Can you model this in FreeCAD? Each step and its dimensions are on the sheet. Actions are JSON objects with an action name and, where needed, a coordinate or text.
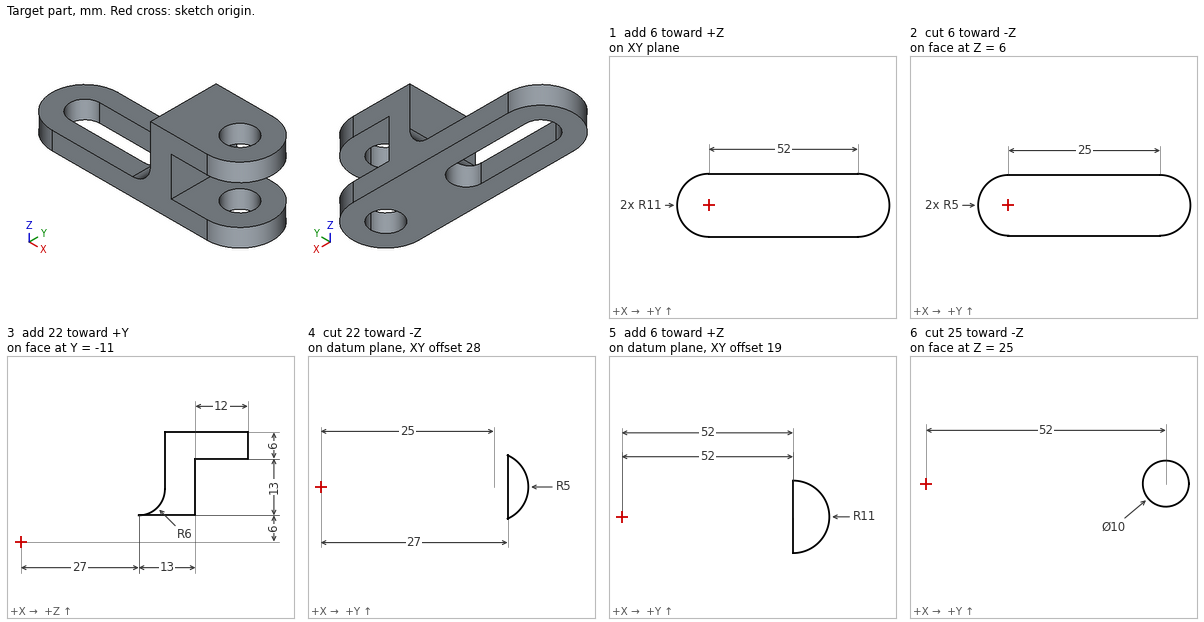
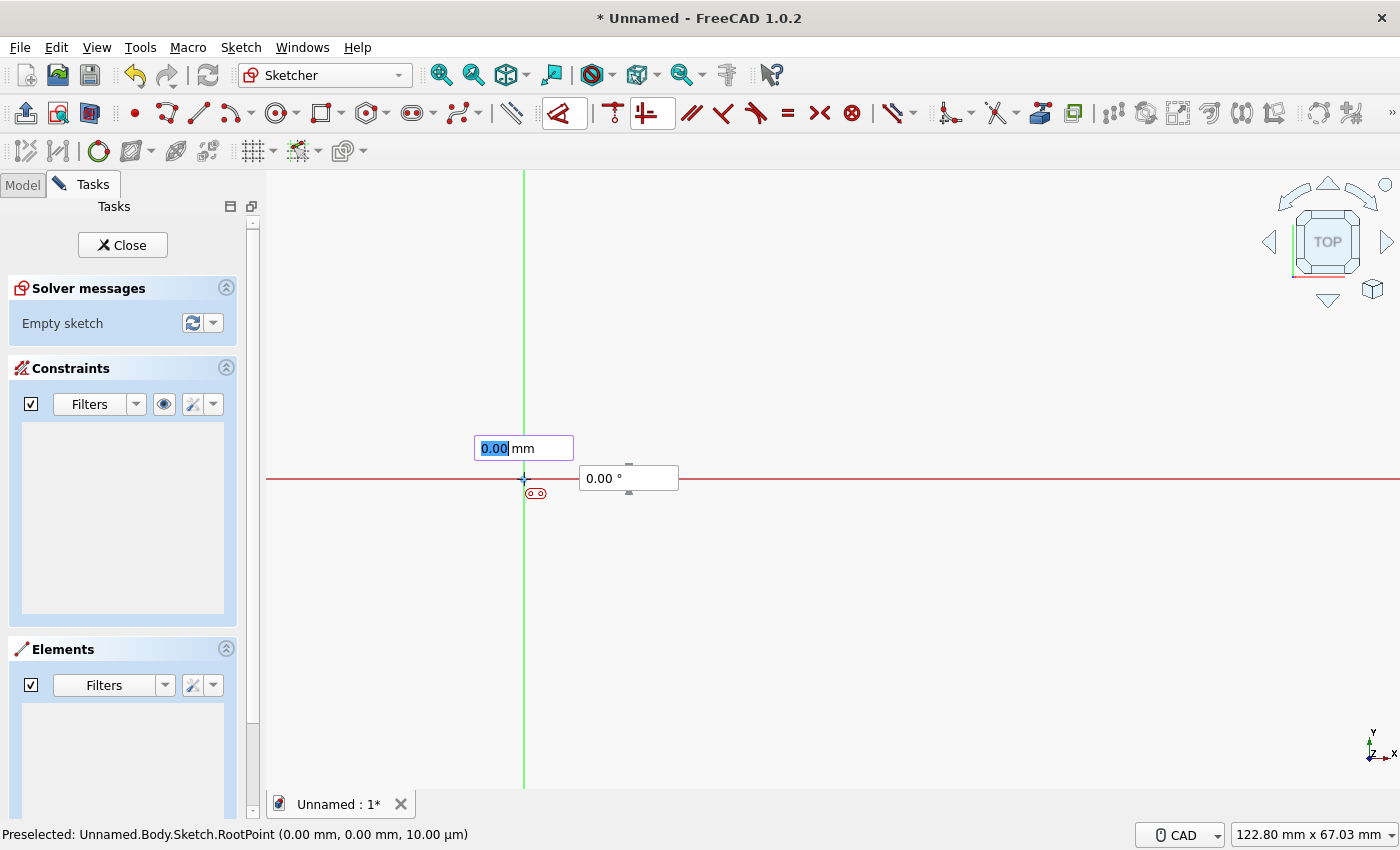
{"action": "left_click", "coordinate": [1004, 470]}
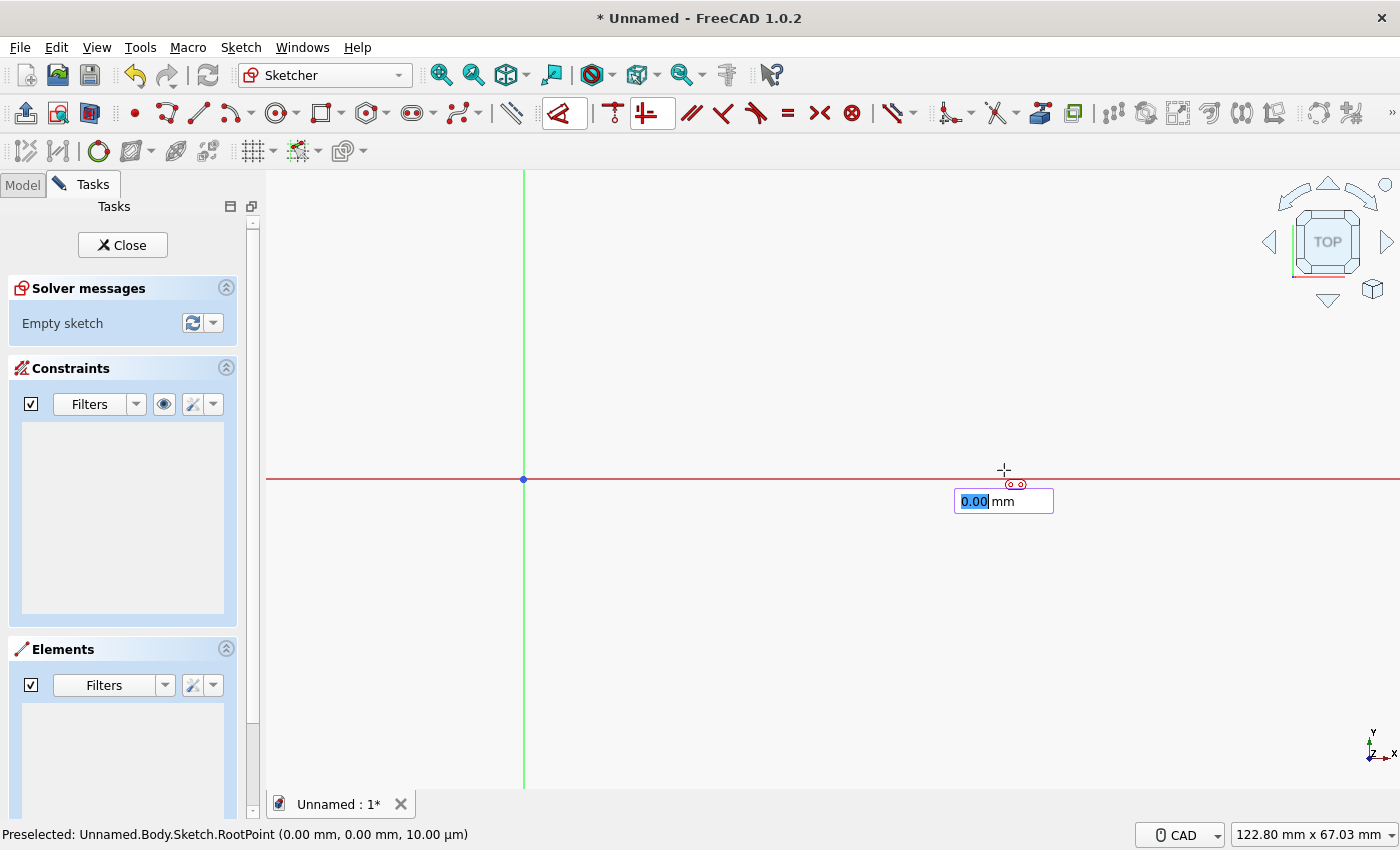
{"action": "left_click", "coordinate": [764, 377]}
{"action": "key", "text": "Escape"}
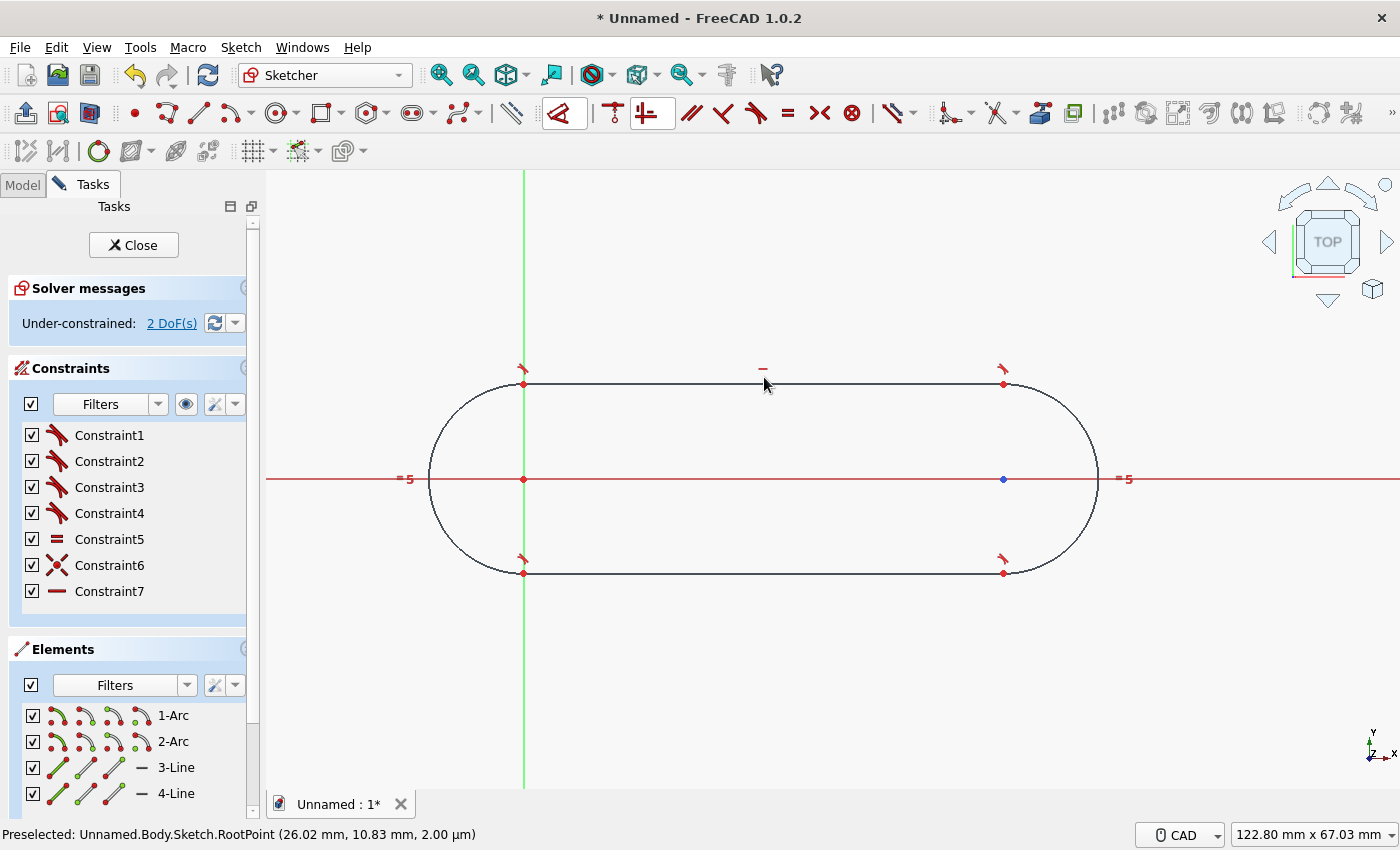
{"action": "left_click", "coordinate": [558, 114]}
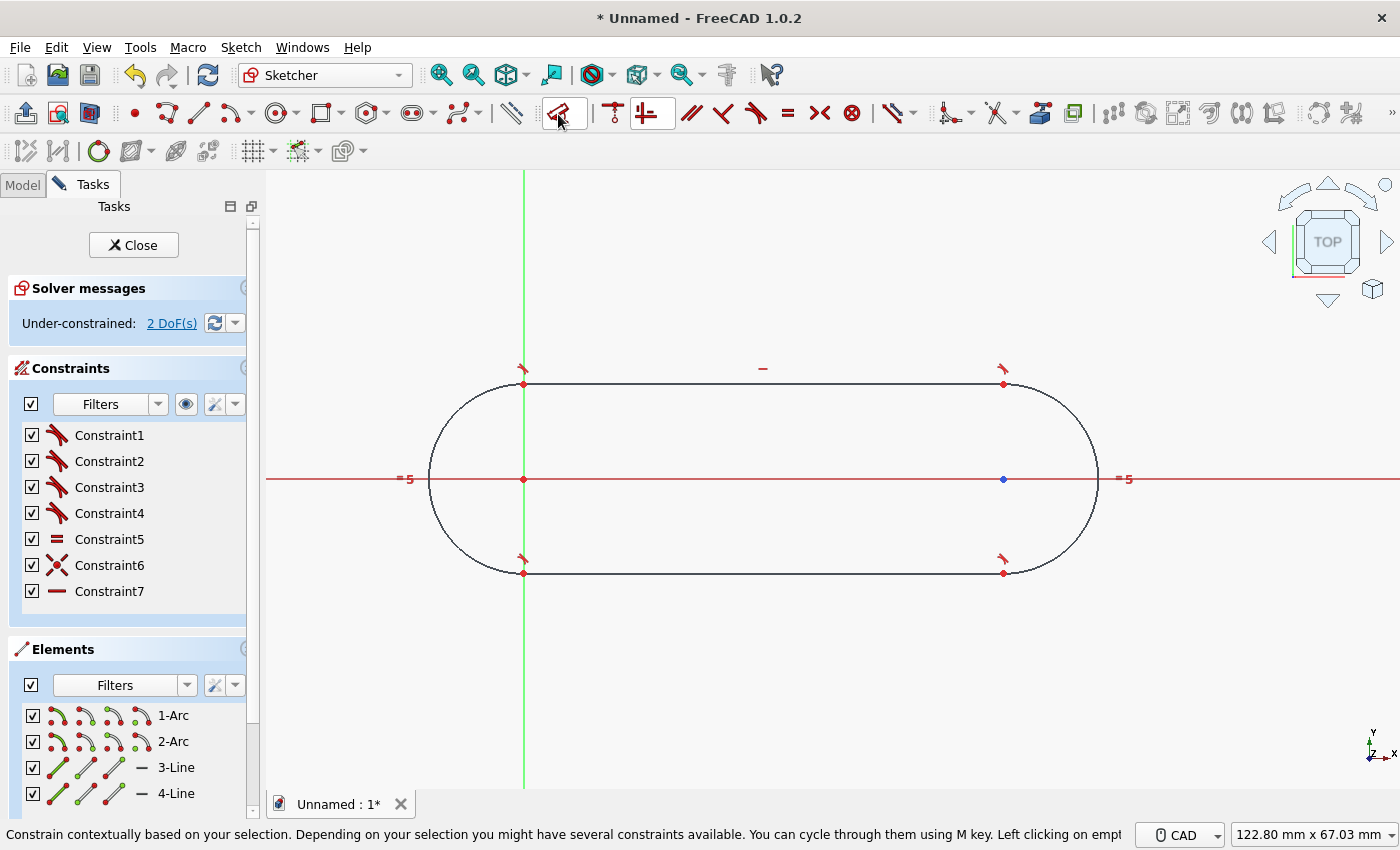
{"action": "left_click", "coordinate": [447, 423]}
{"action": "left_click", "coordinate": [421, 404]}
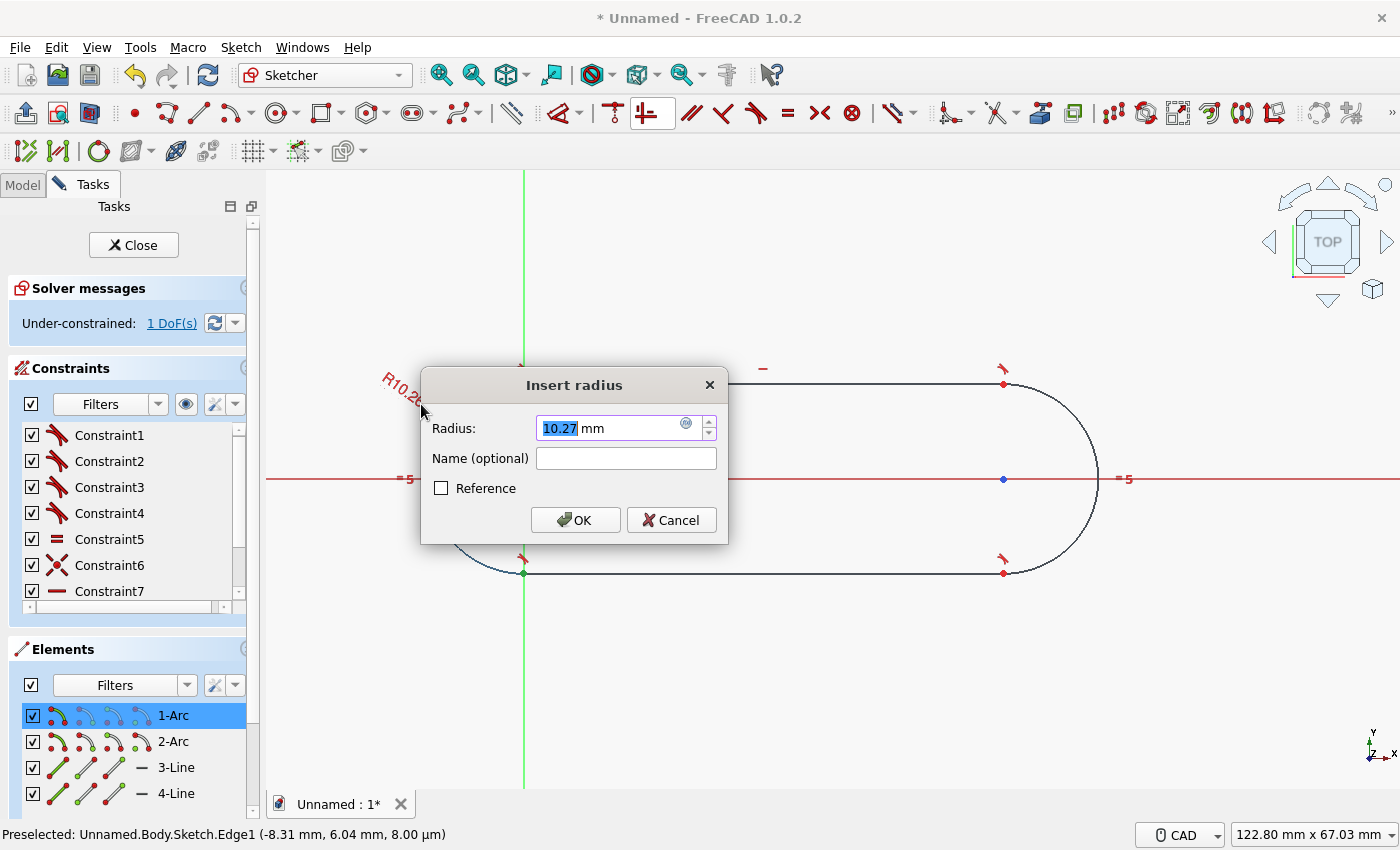
{"action": "type", "text": "11"}
{"action": "key", "text": "Return"}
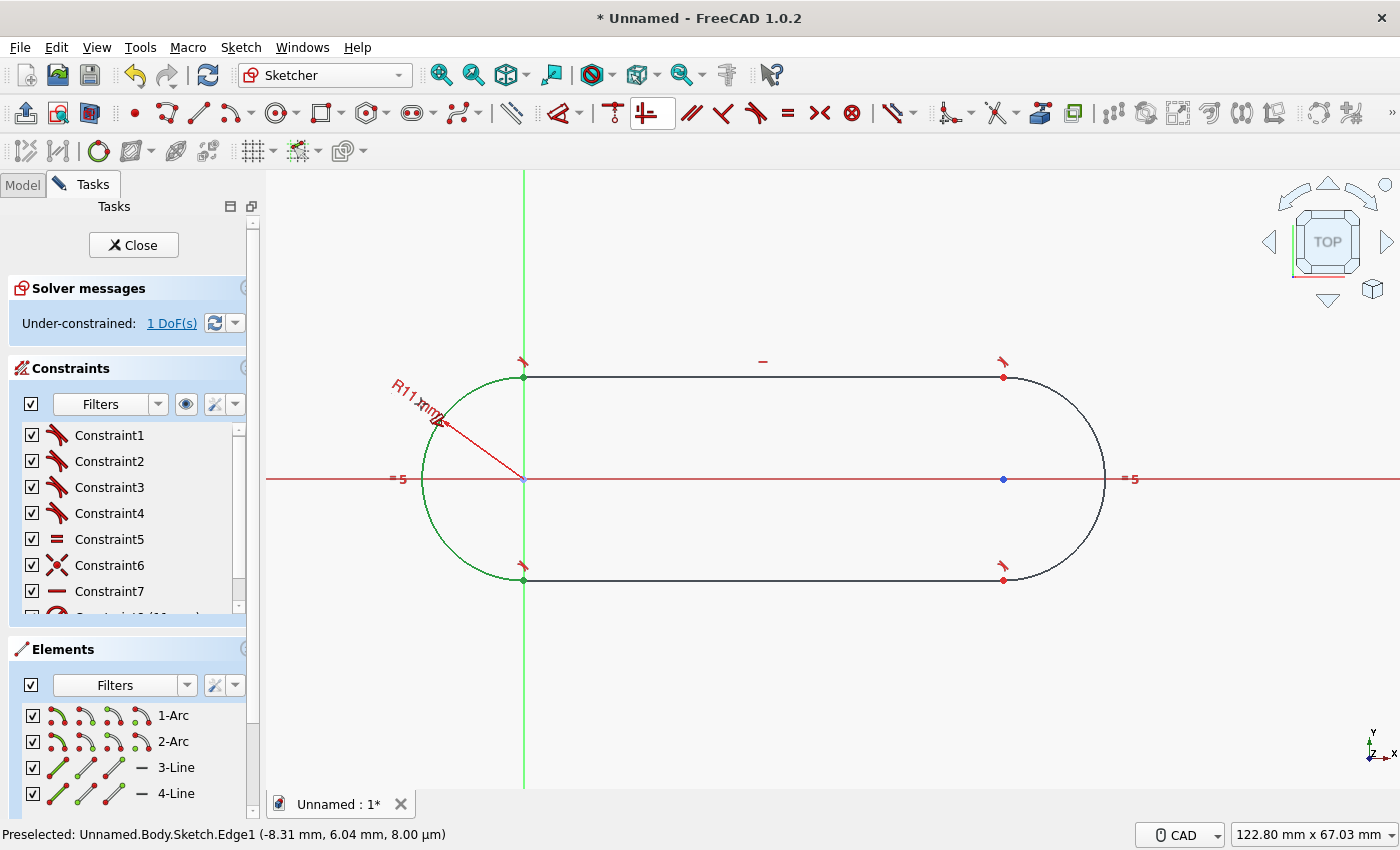
{"action": "left_click", "coordinate": [668, 377]}
{"action": "left_click", "coordinate": [764, 343]}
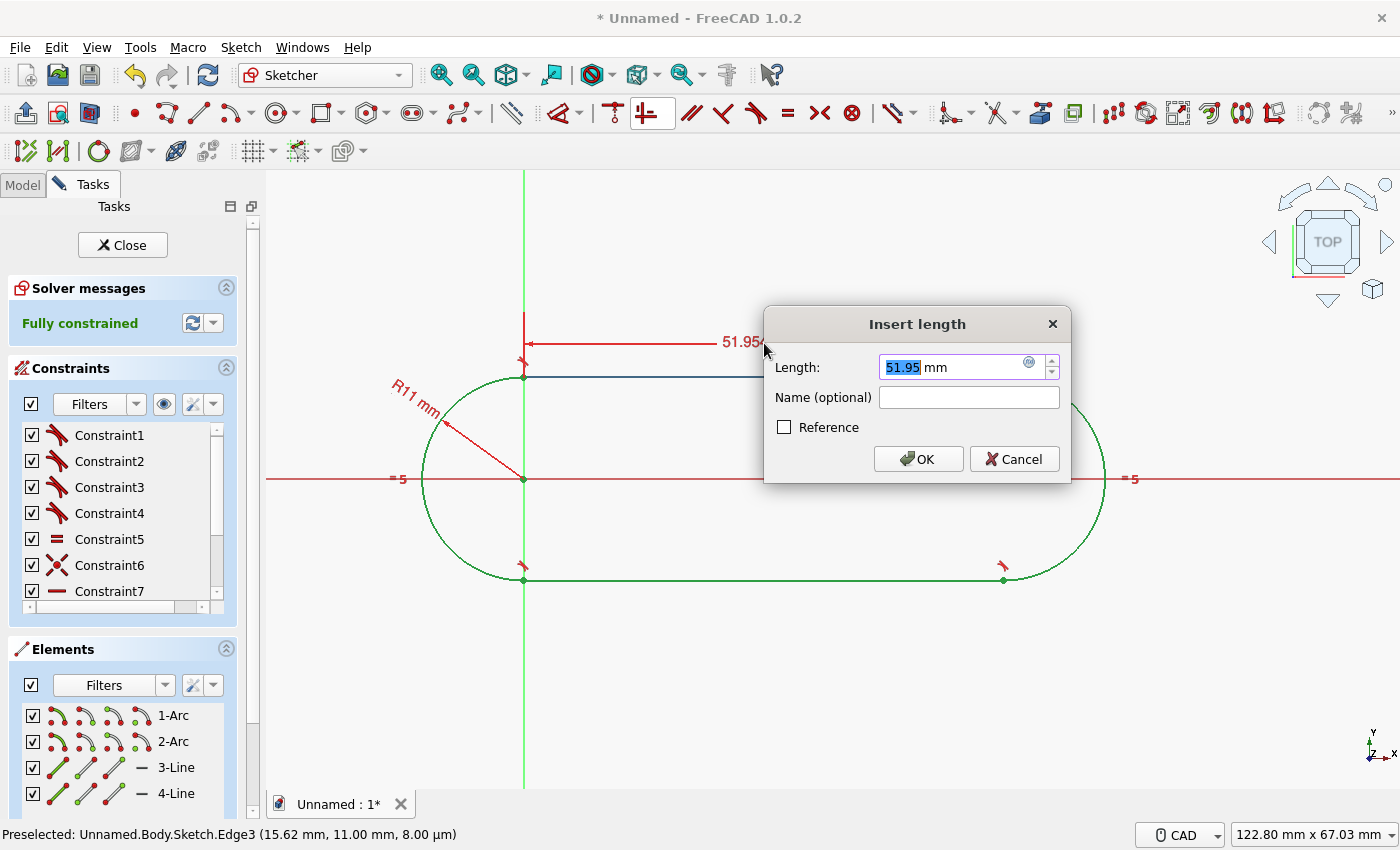
{"action": "type", "text": "52"}
{"action": "key", "text": "Return"}
{"action": "key", "text": "Escape"}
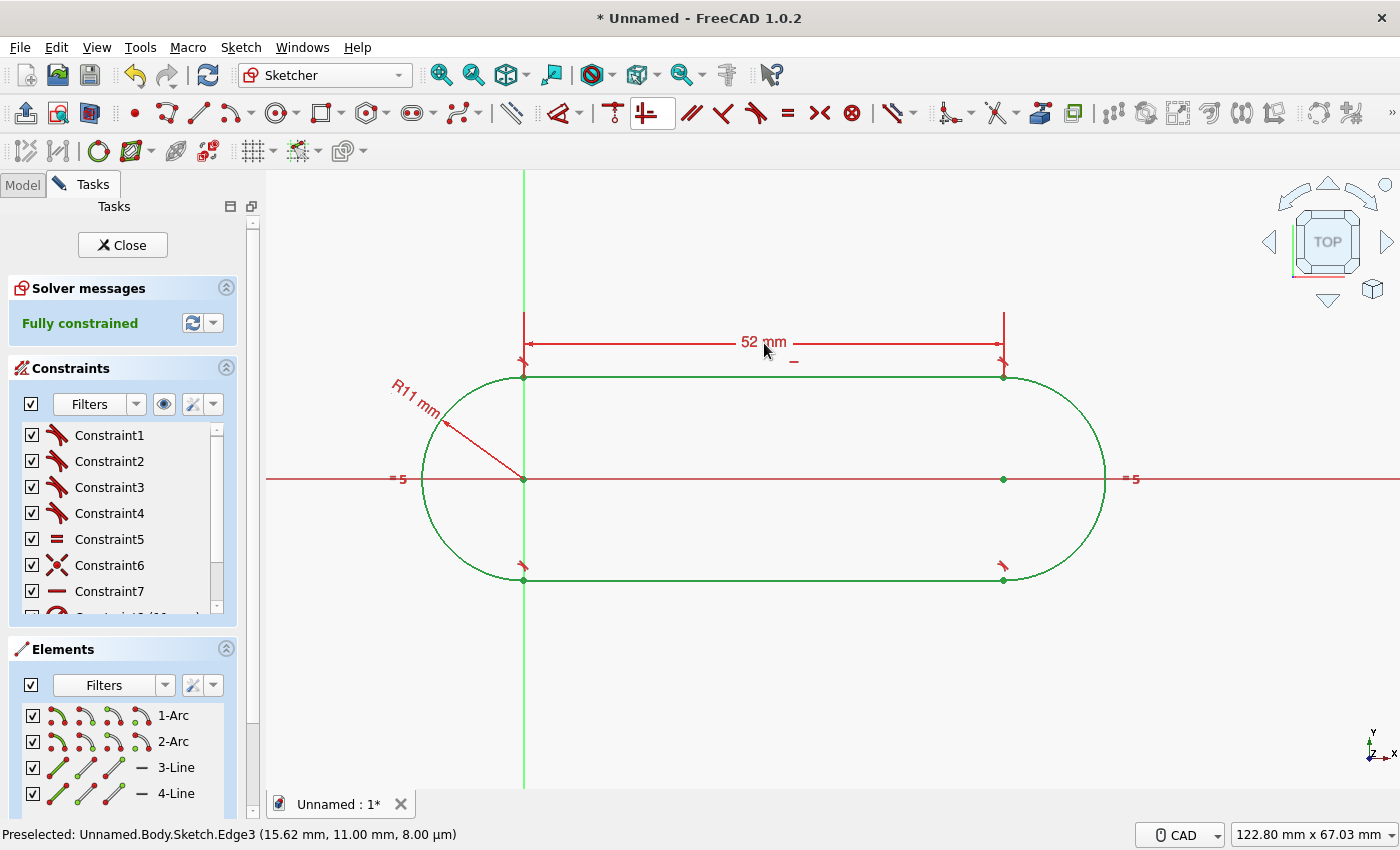
{"action": "left_click", "coordinate": [123, 245]}